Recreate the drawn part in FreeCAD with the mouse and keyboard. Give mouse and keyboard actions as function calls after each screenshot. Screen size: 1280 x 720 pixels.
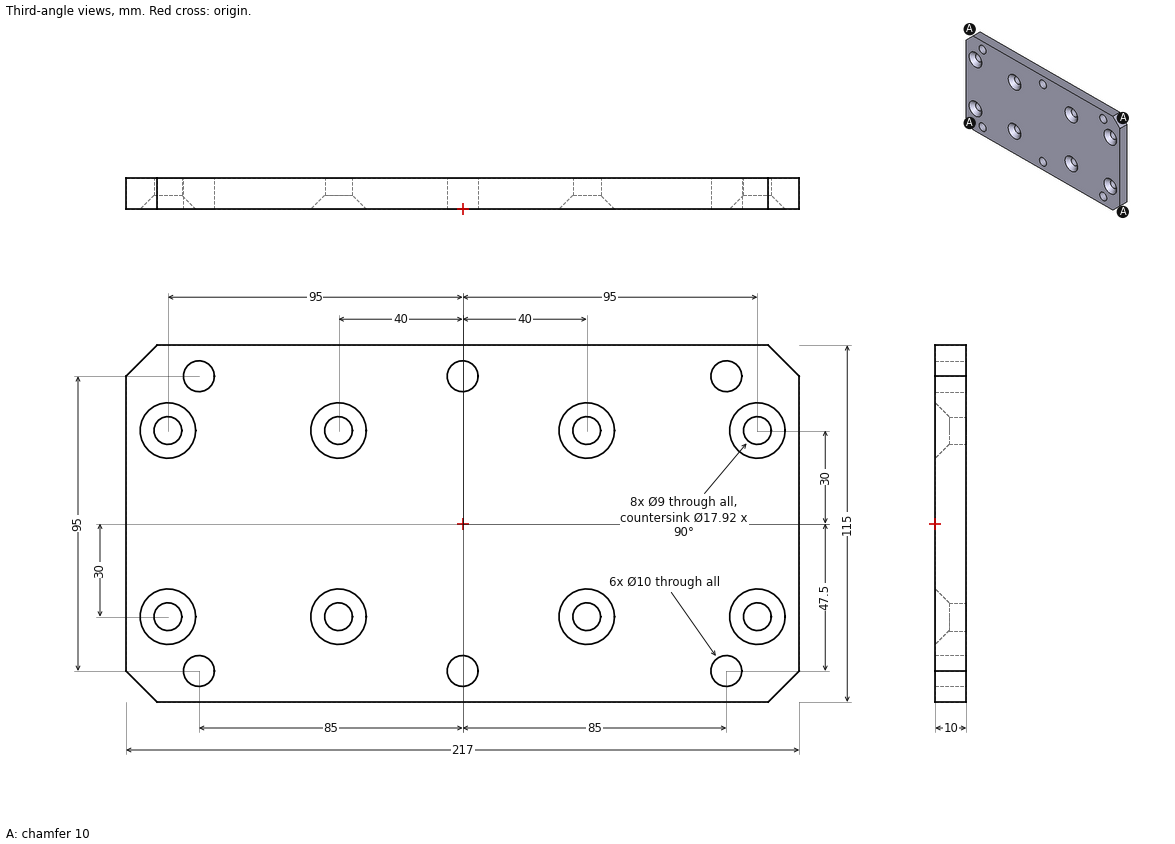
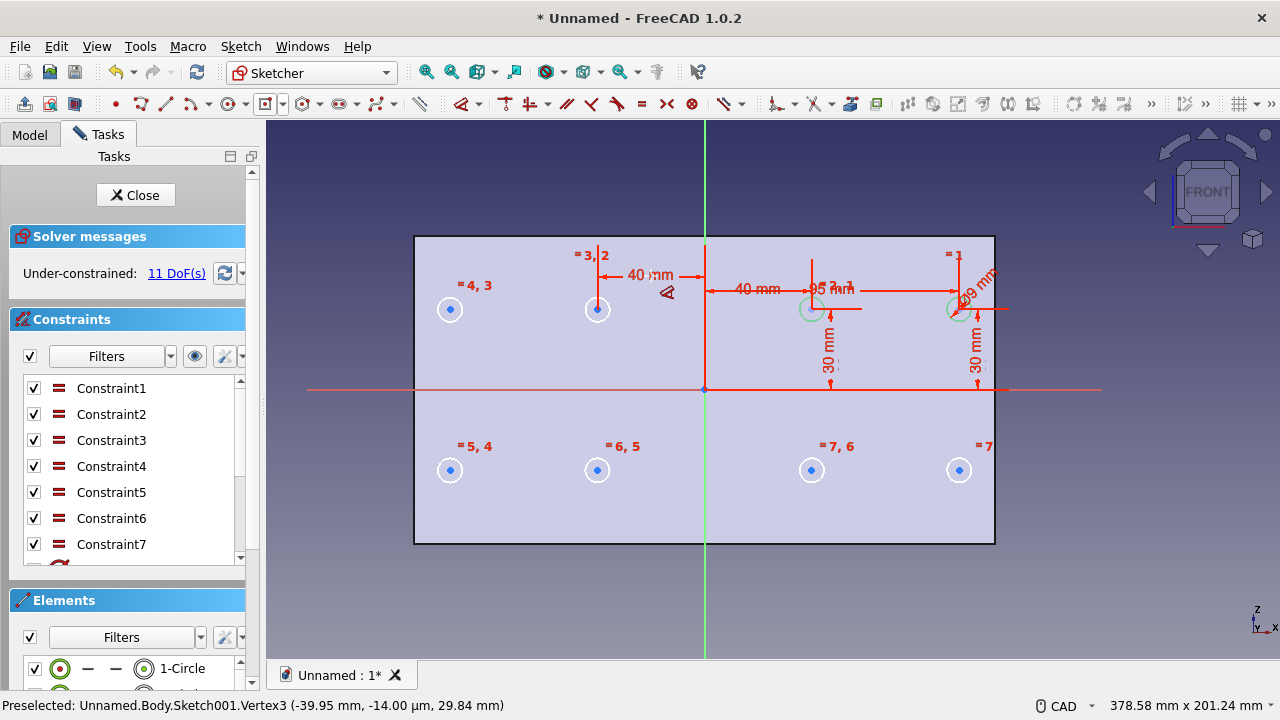
click(598, 310)
click(564, 350)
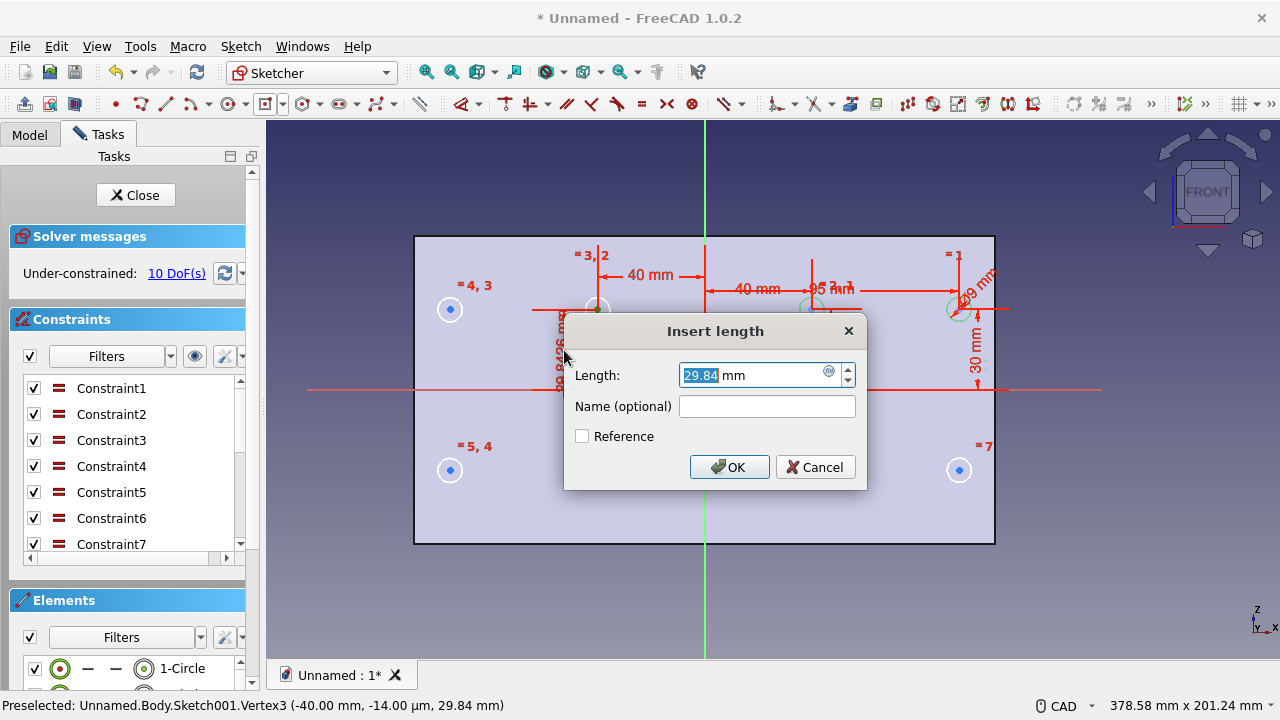
text(30)
key(Return)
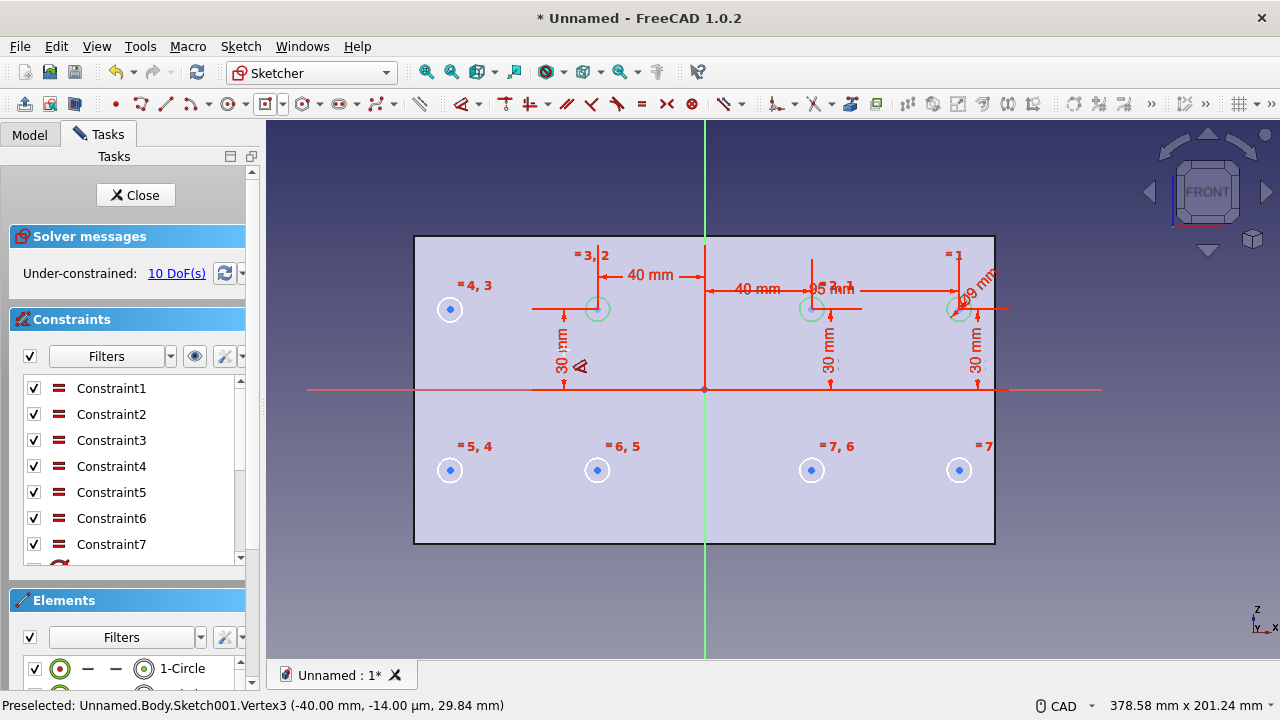
click(450, 310)
click(577, 276)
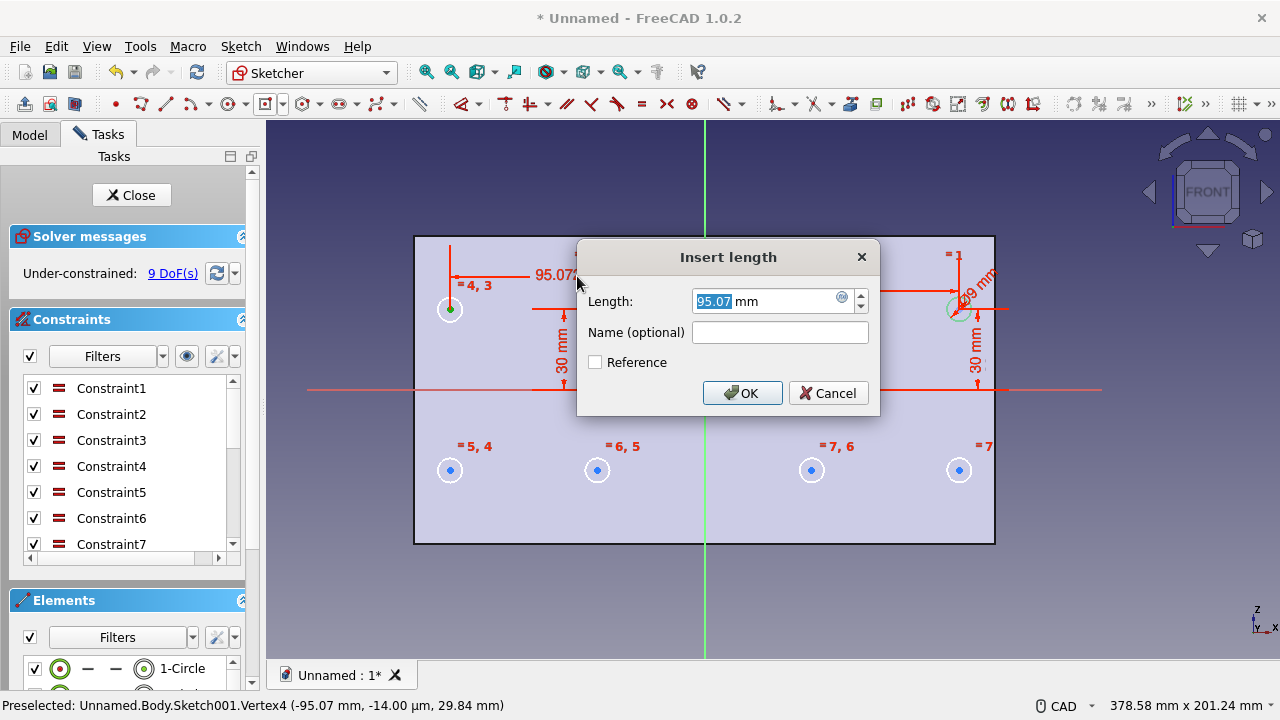
text(95)
key(Return)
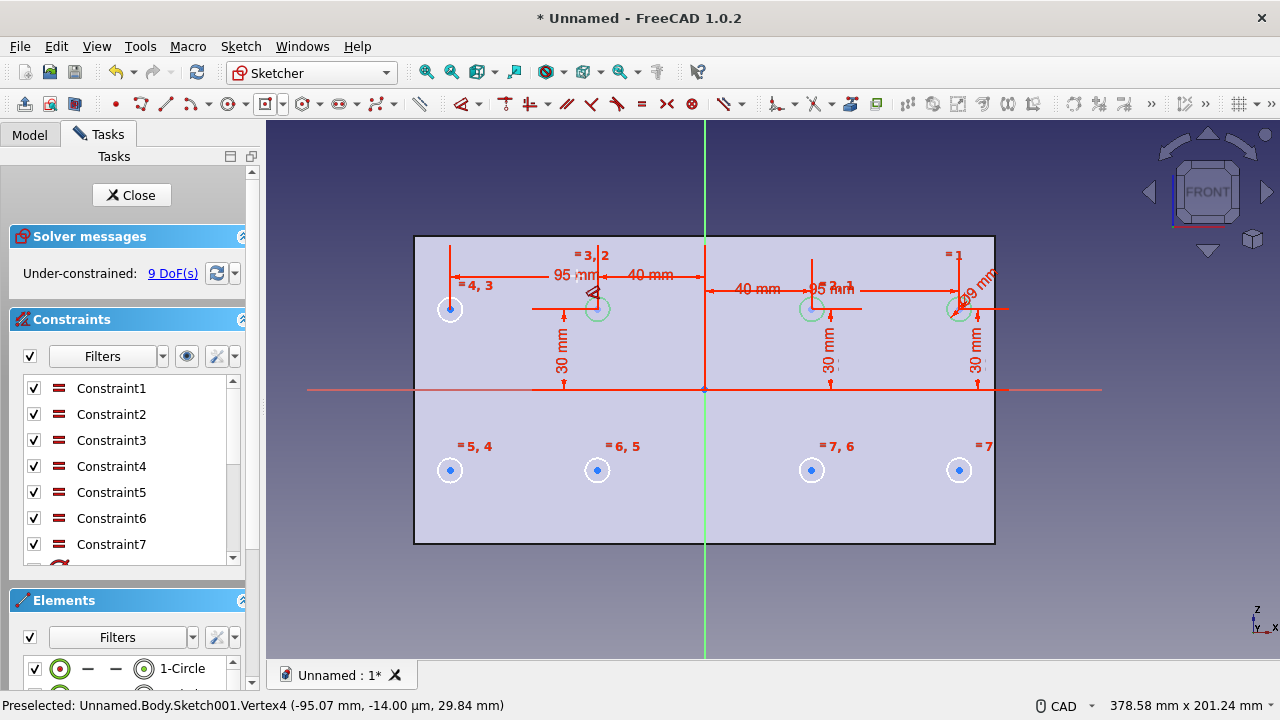
click(450, 310)
click(416, 350)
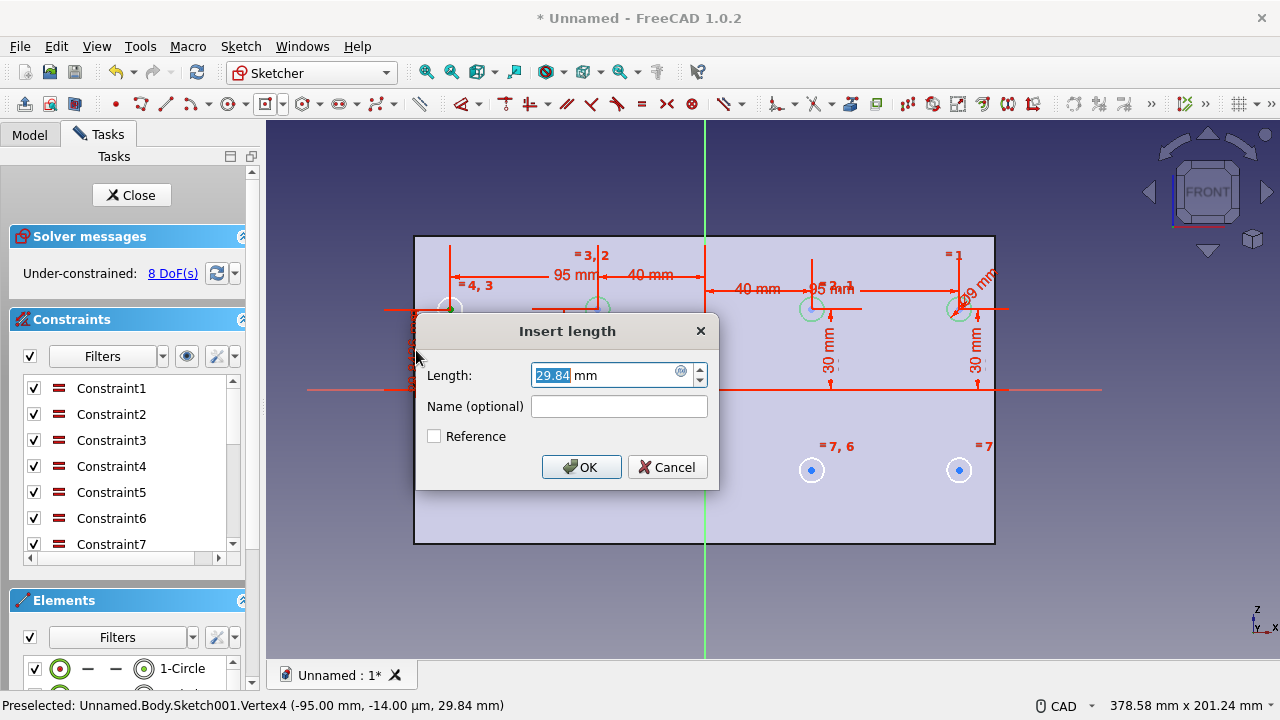
text(30)
key(Return)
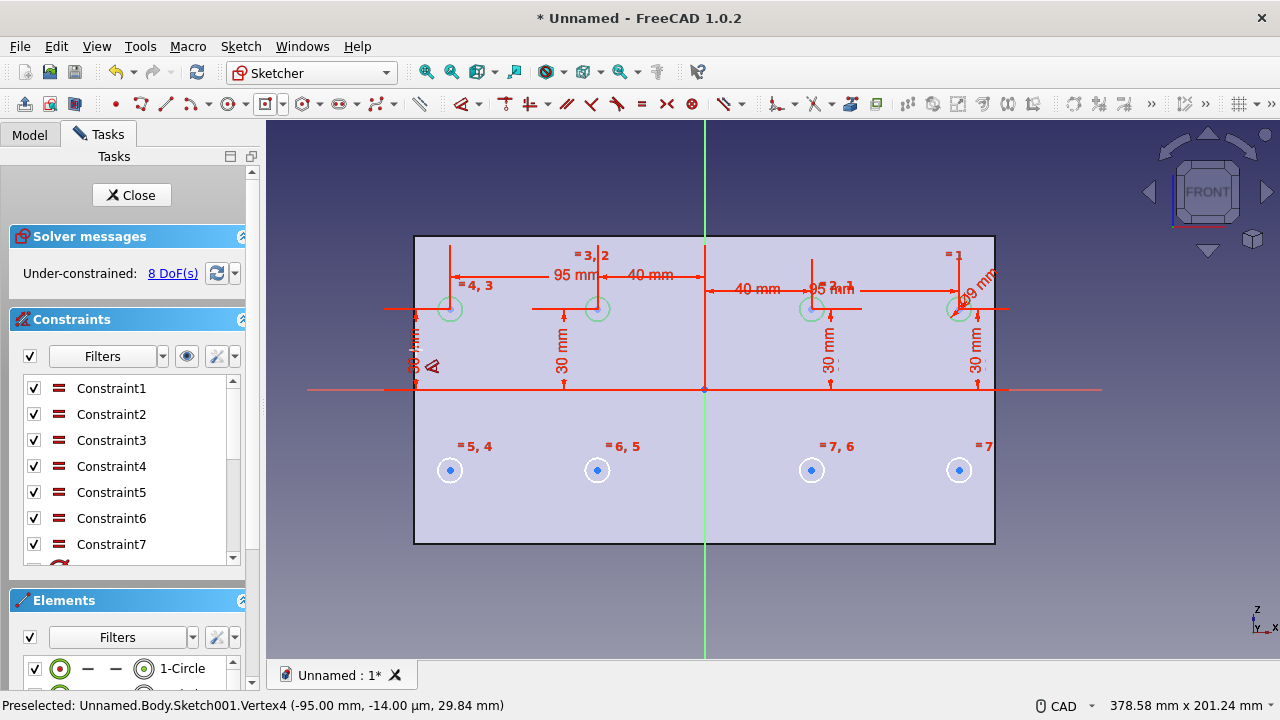
click(450, 470)
click(577, 504)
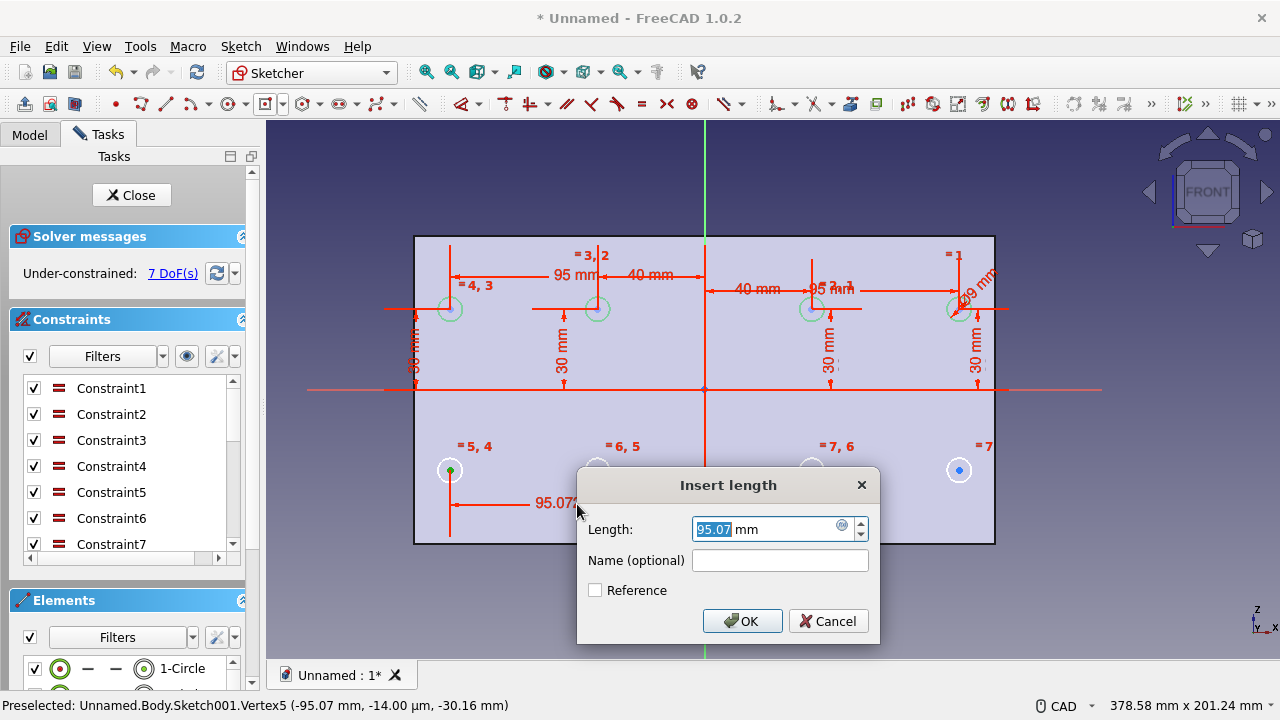
text(95)
key(Return)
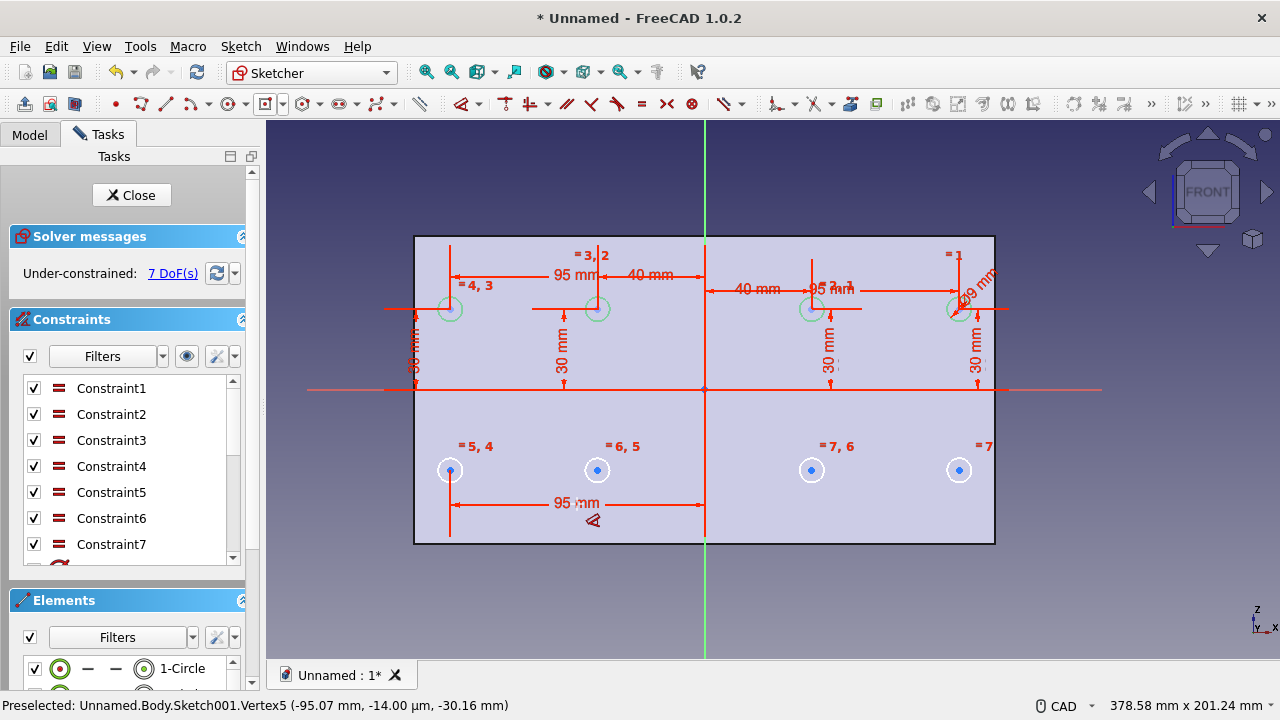
click(450, 470)
click(416, 430)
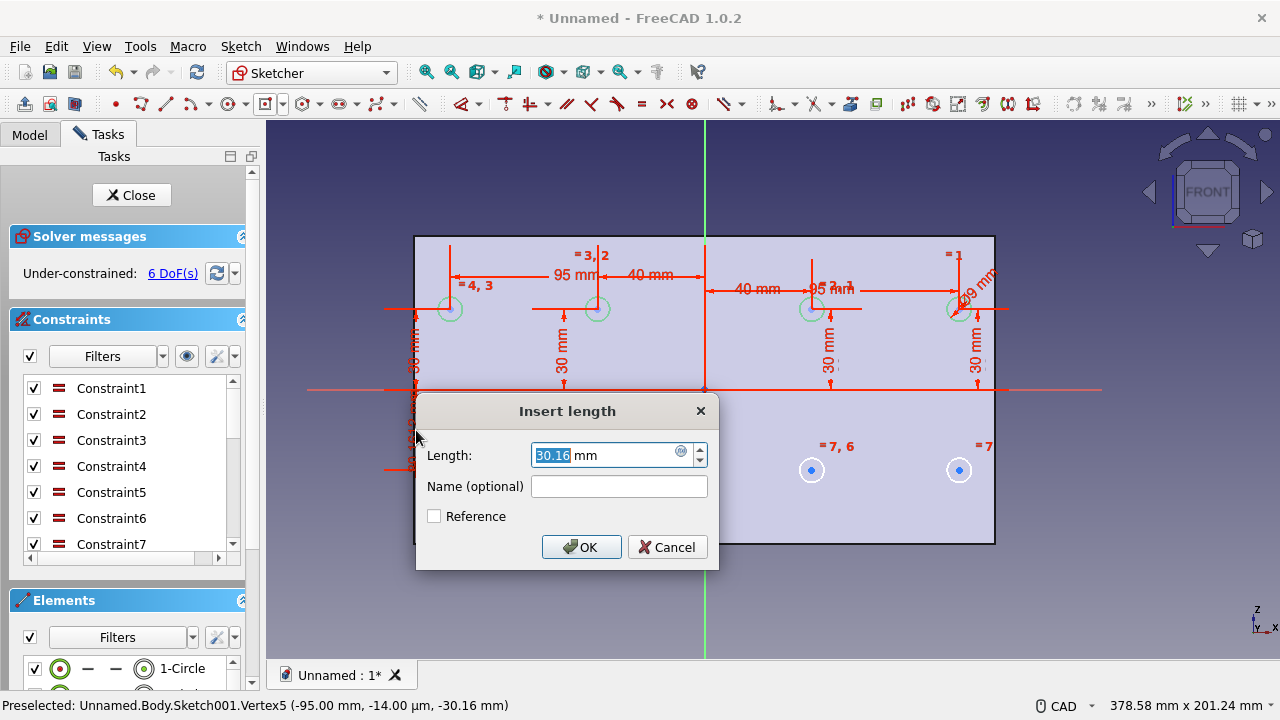
text(30)
key(Return)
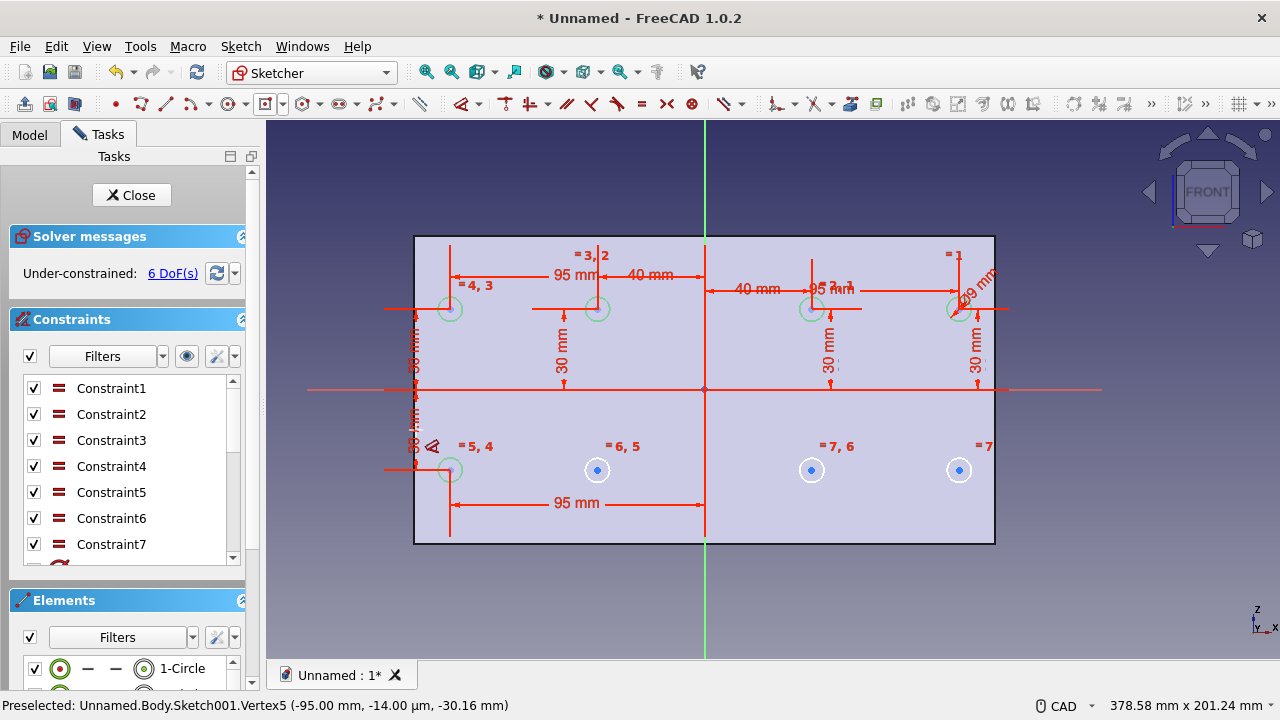
click(597, 470)
click(651, 504)